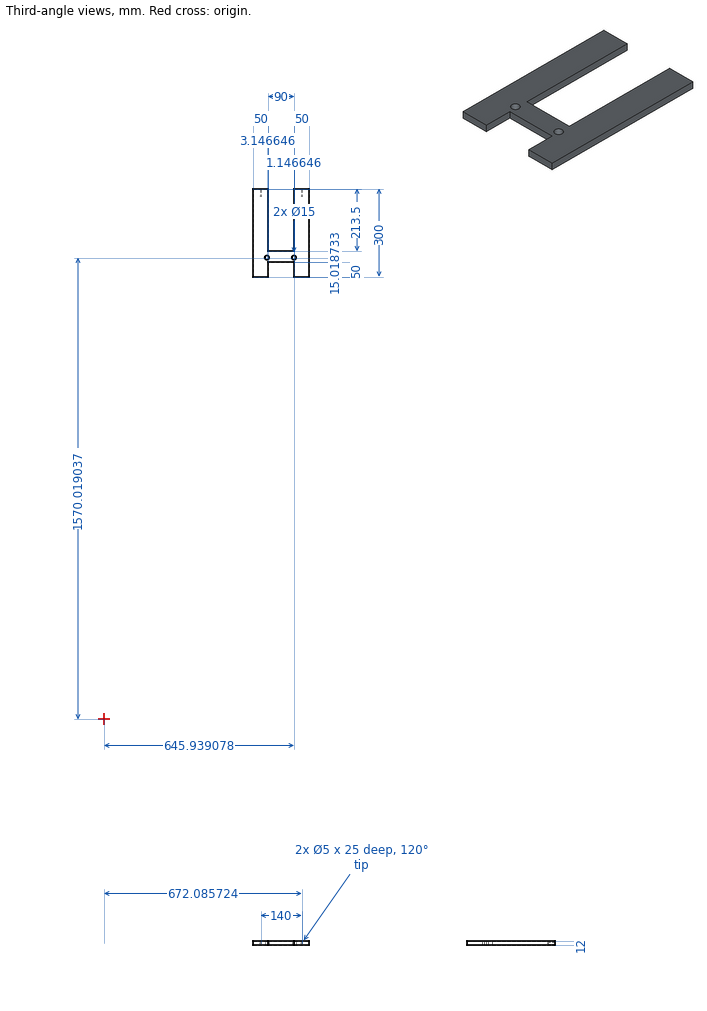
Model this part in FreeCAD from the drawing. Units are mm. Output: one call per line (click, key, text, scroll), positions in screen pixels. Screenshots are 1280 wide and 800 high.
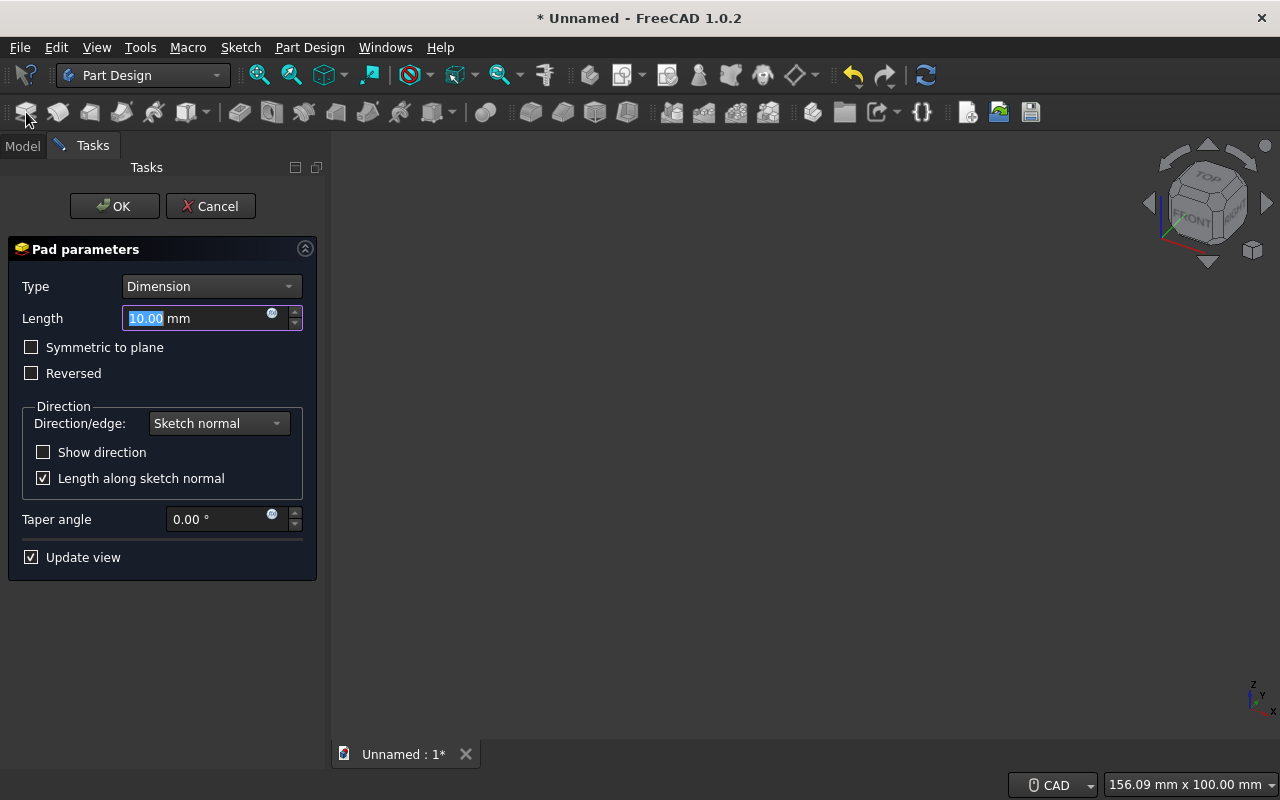
text(12)
key(Tab)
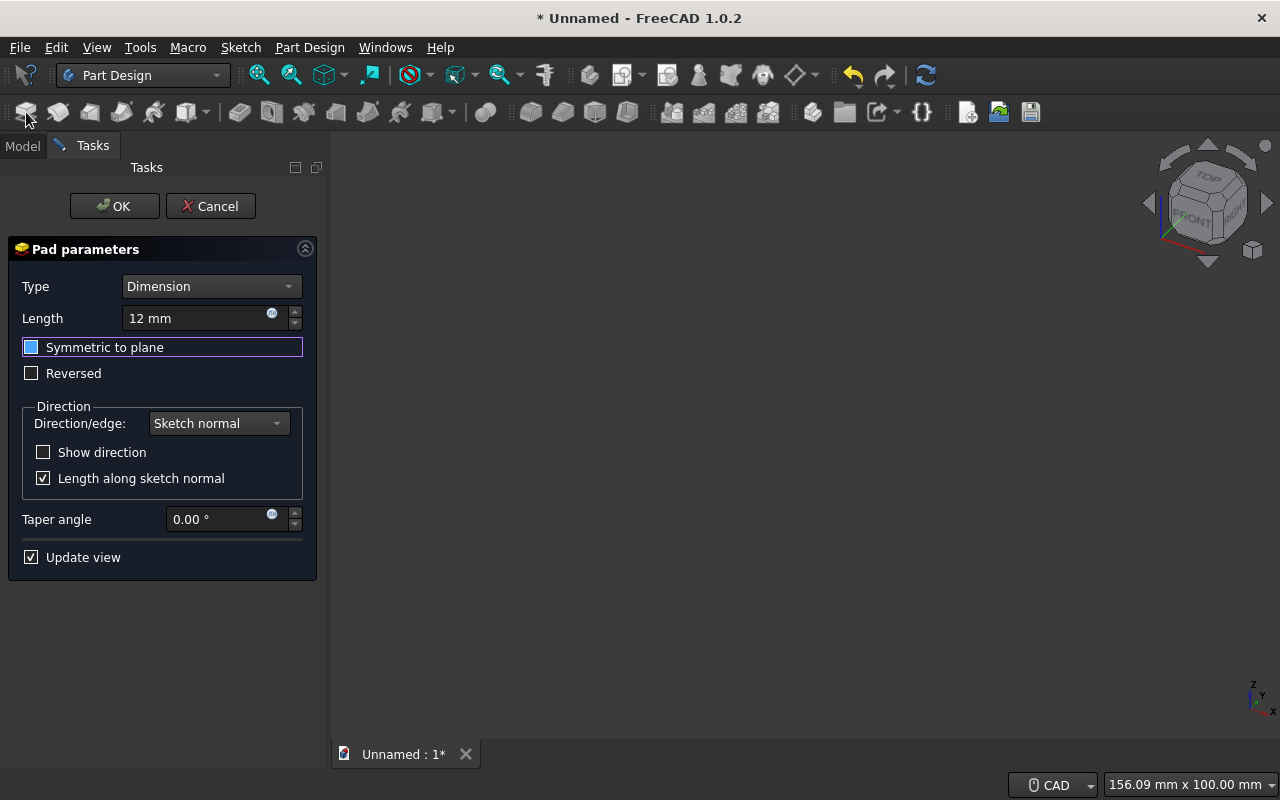
click(30, 347)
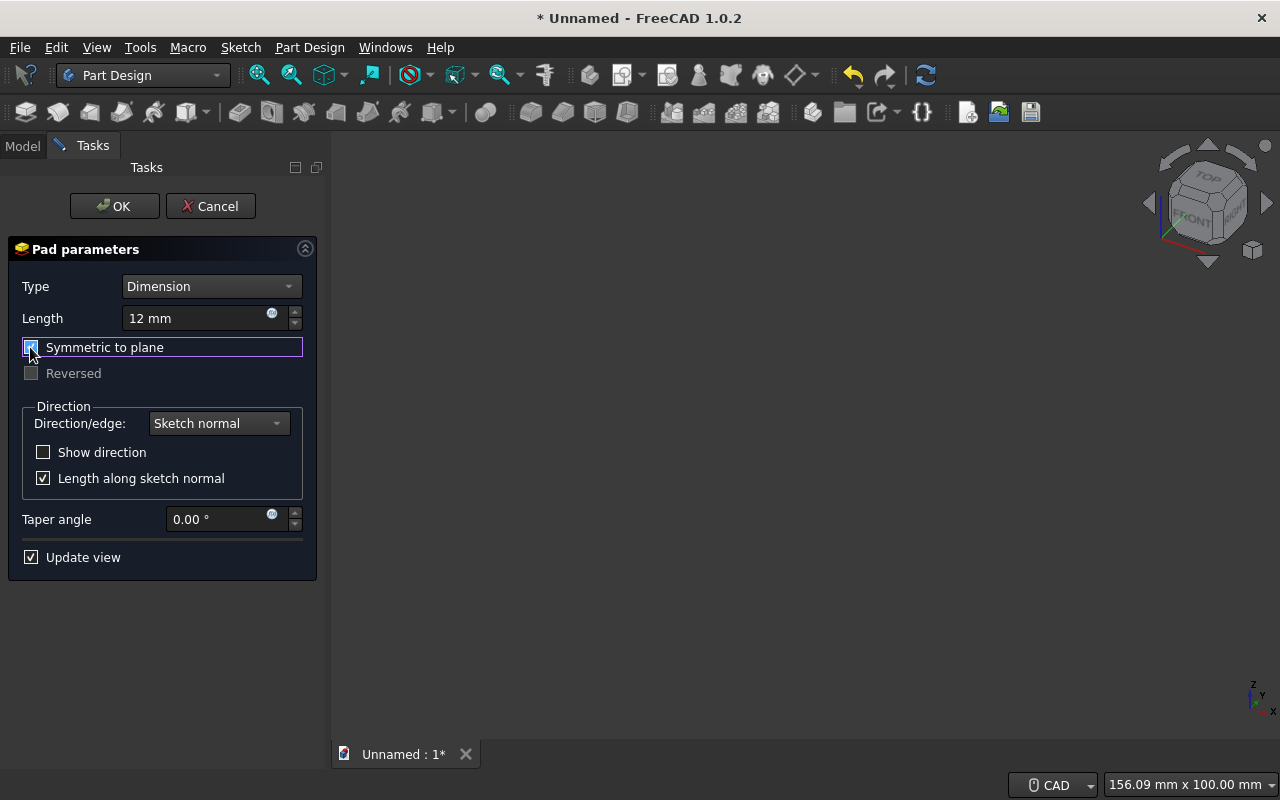
click(115, 206)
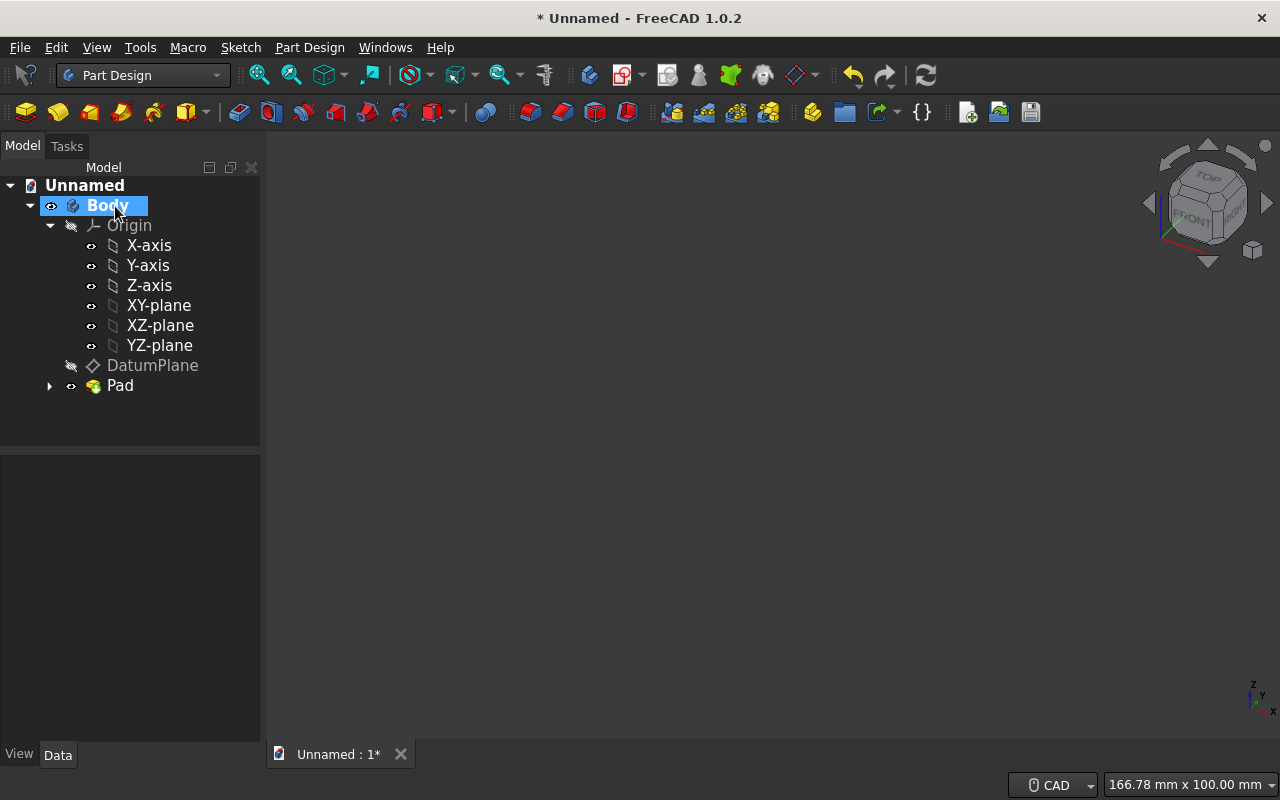
key(v)
key(f)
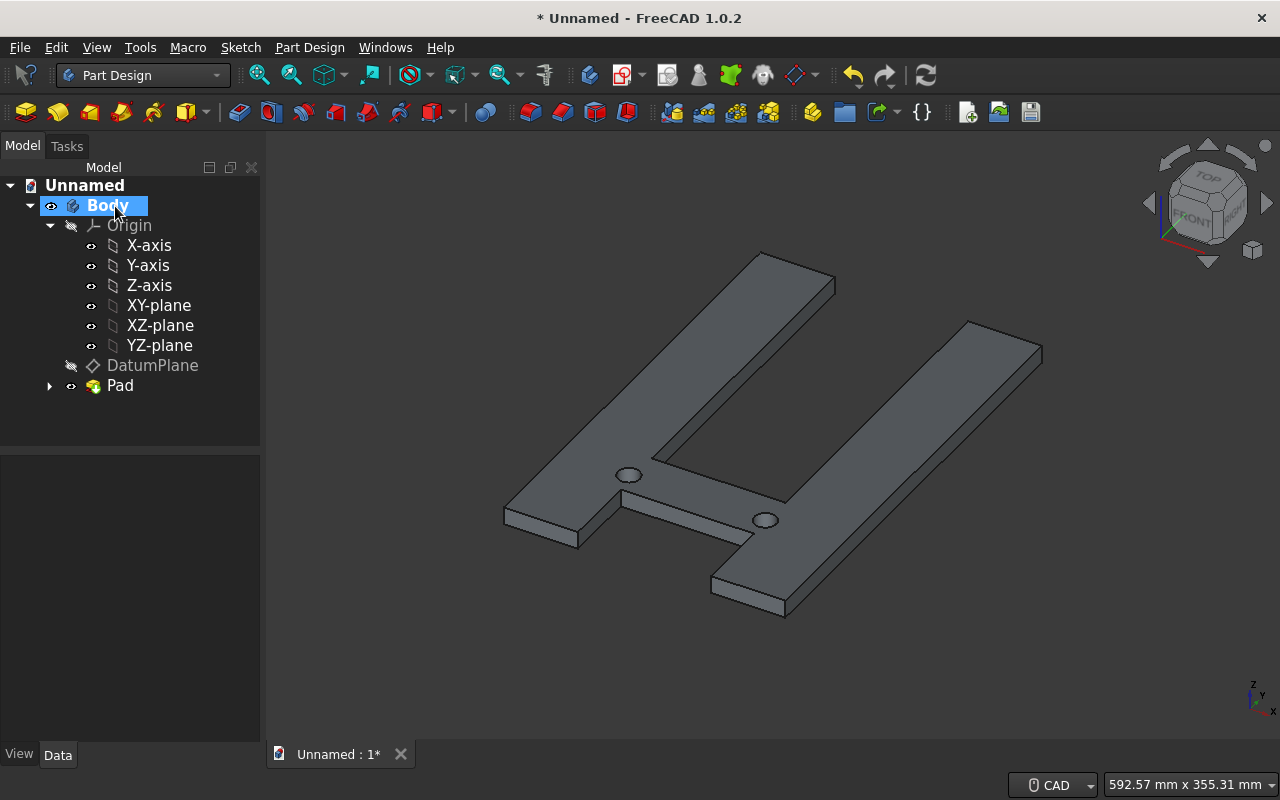
key(4)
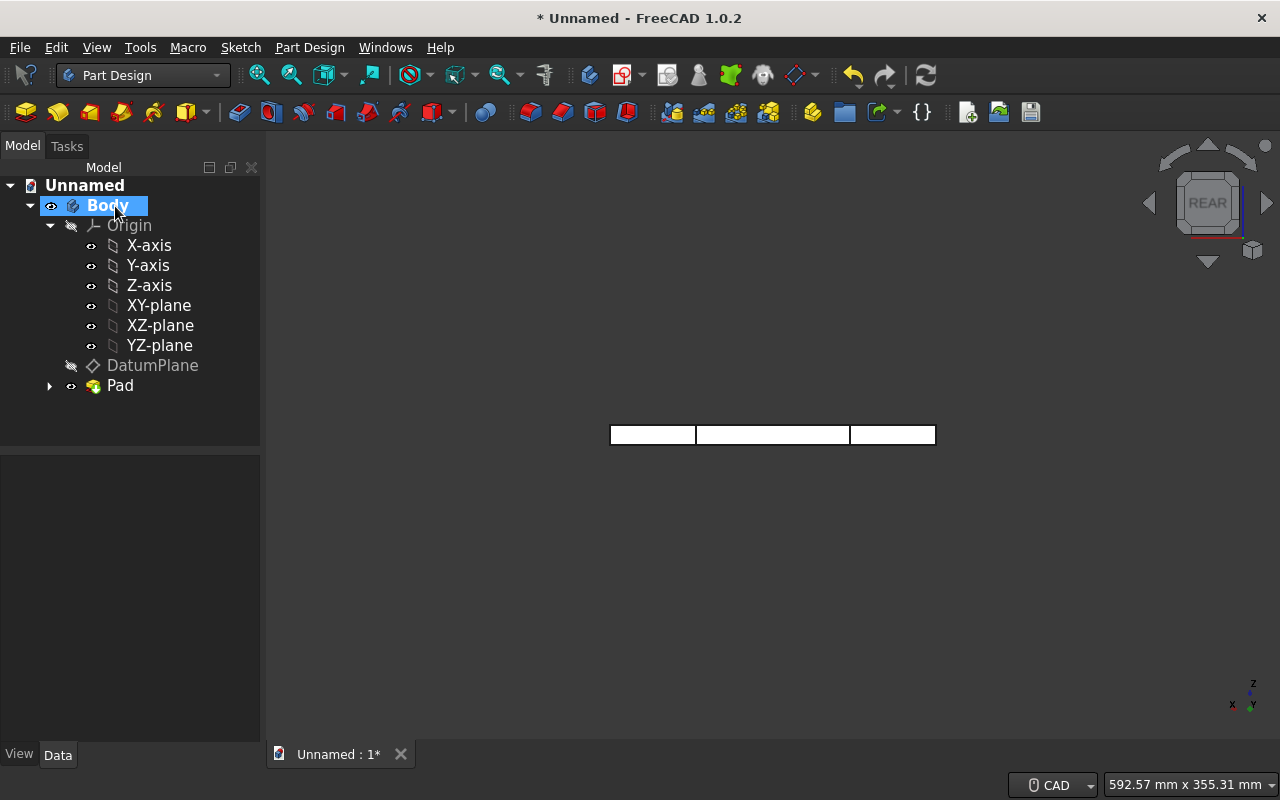
click(260, 76)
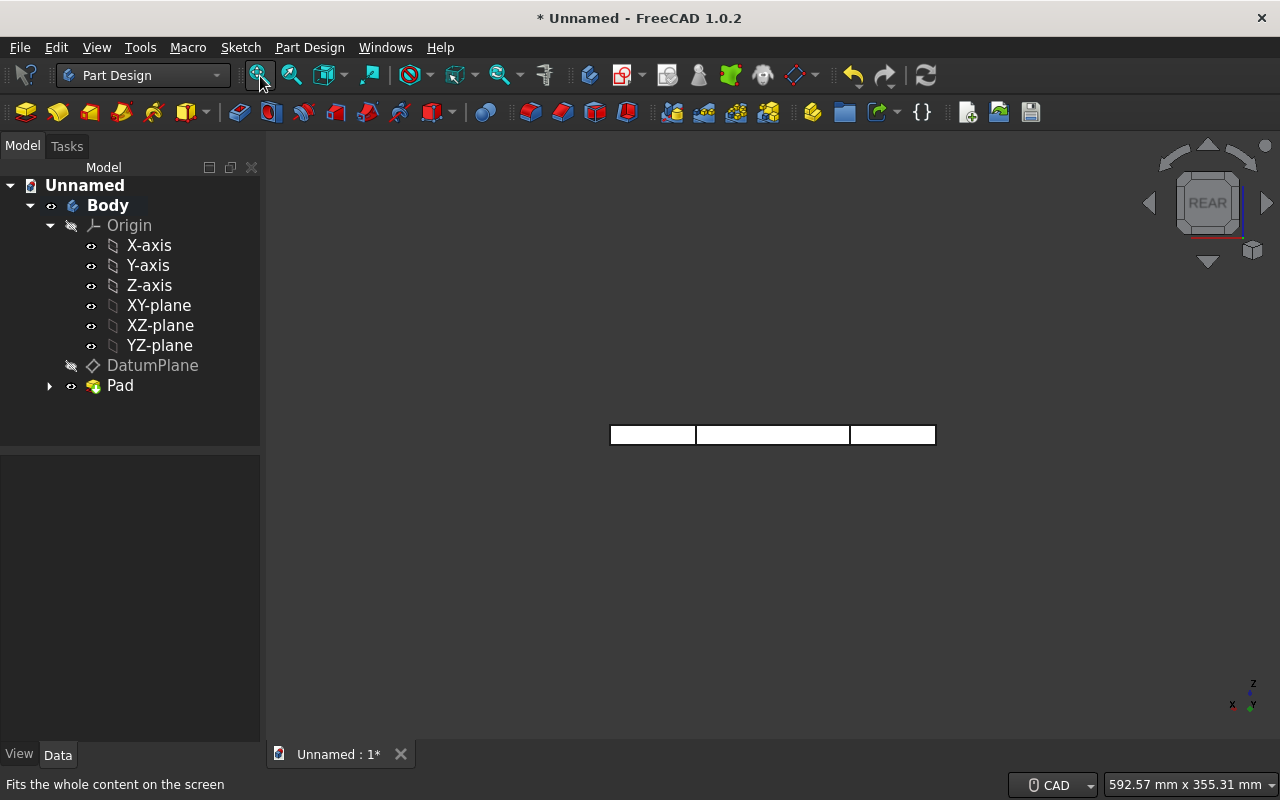
click(868, 434)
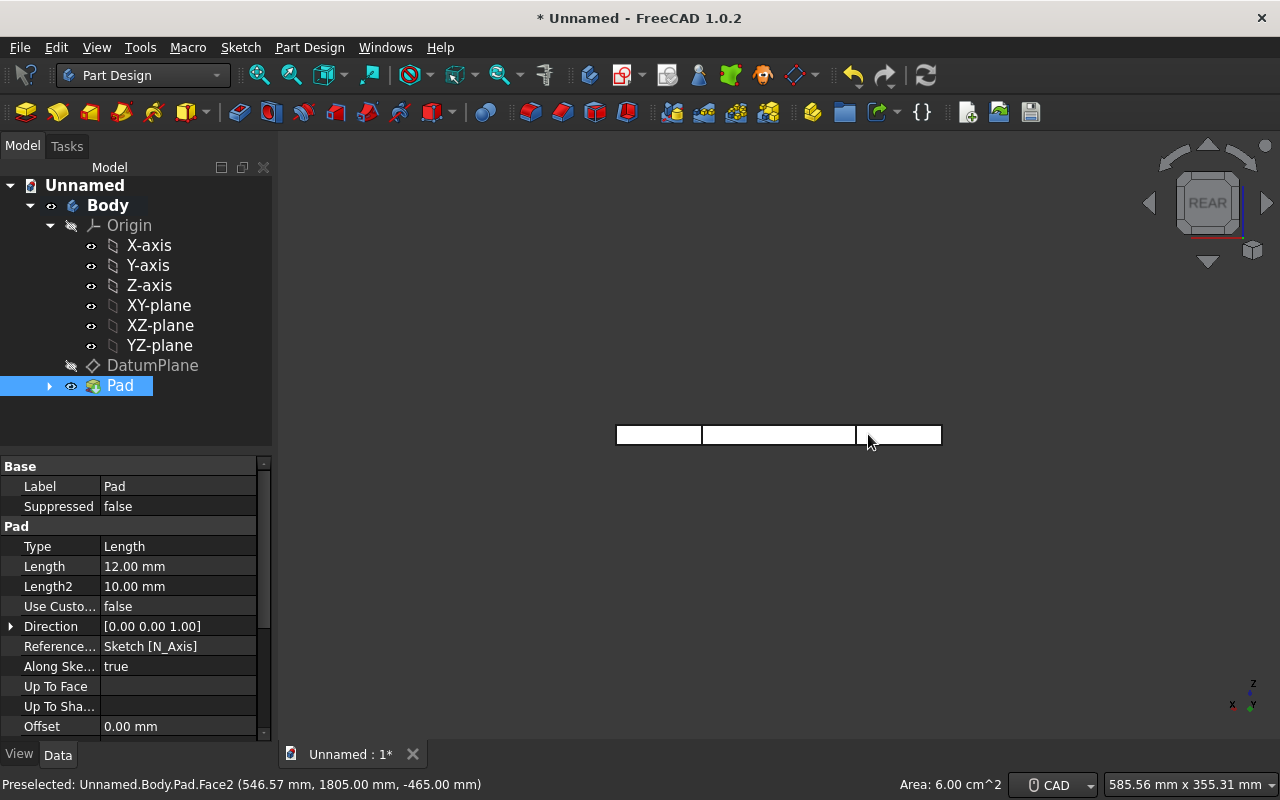
click(622, 76)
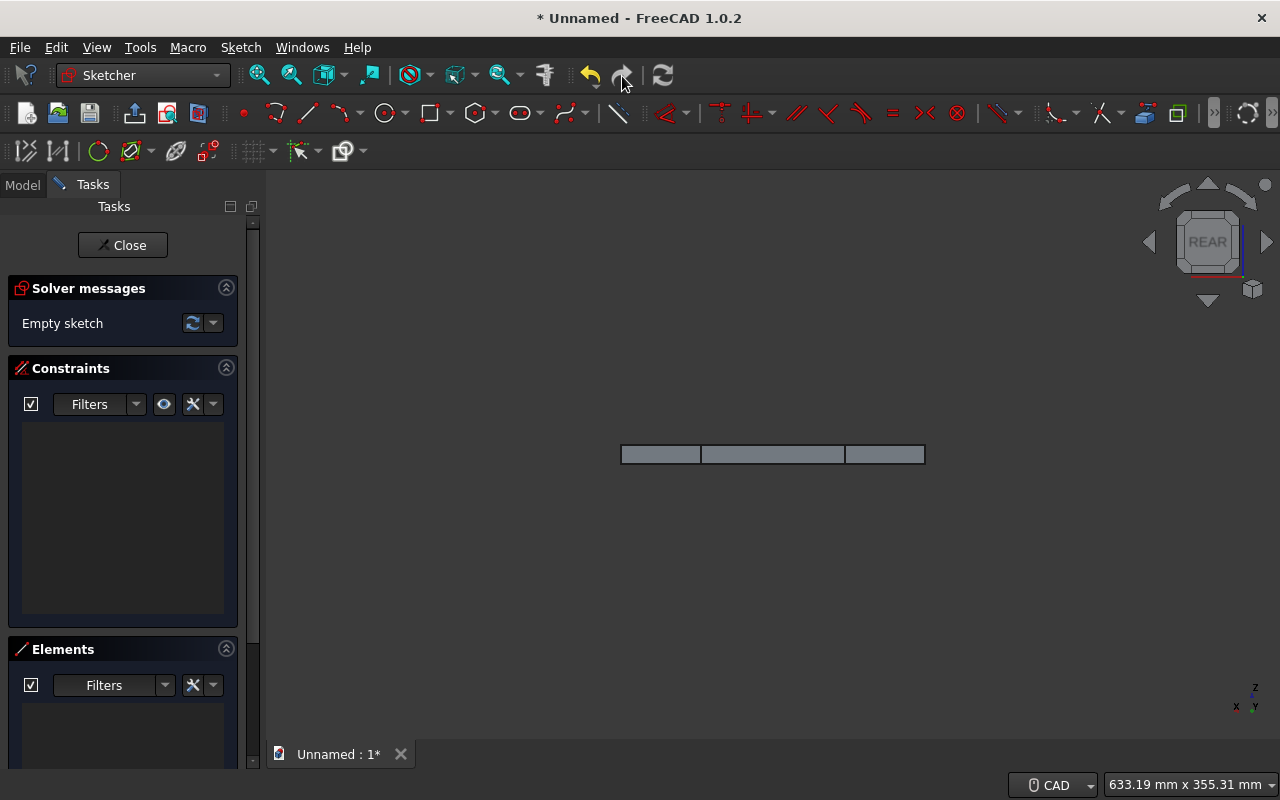
scroll(813, 454, up, 5)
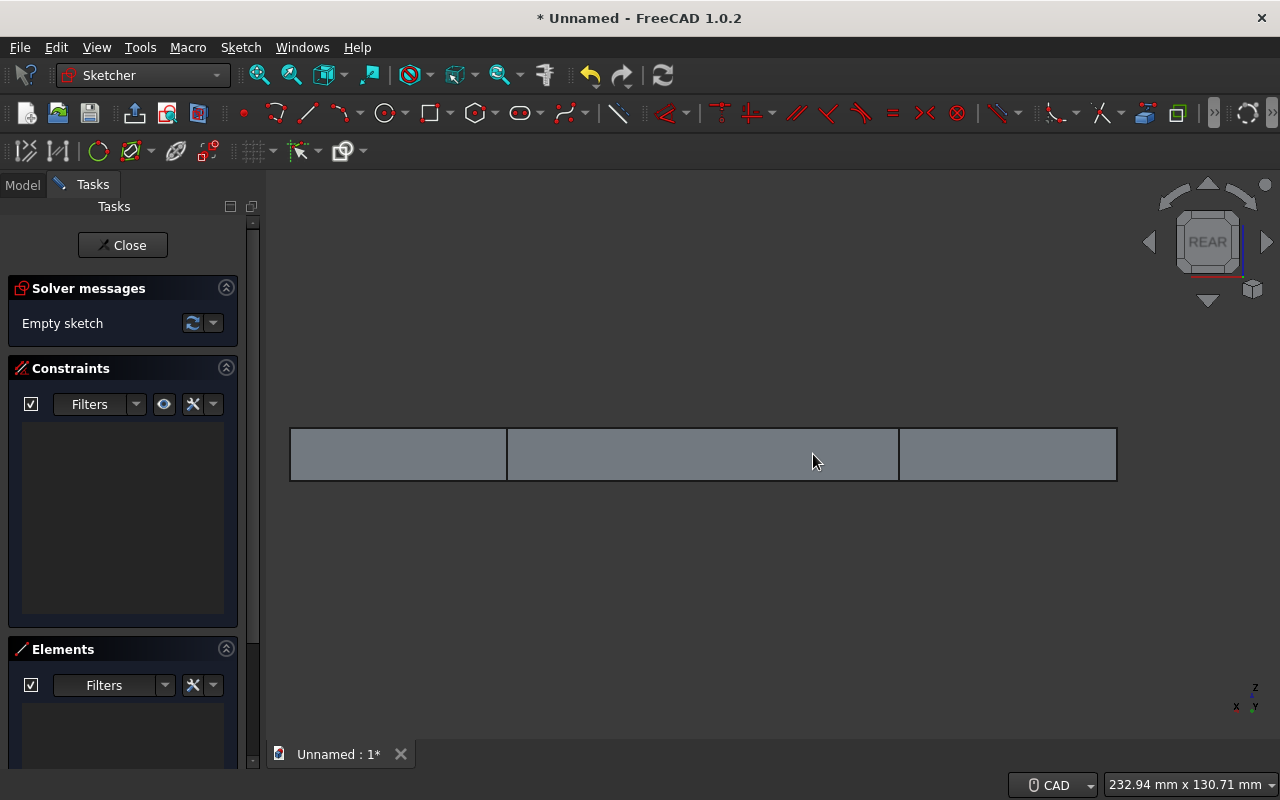
click(386, 114)